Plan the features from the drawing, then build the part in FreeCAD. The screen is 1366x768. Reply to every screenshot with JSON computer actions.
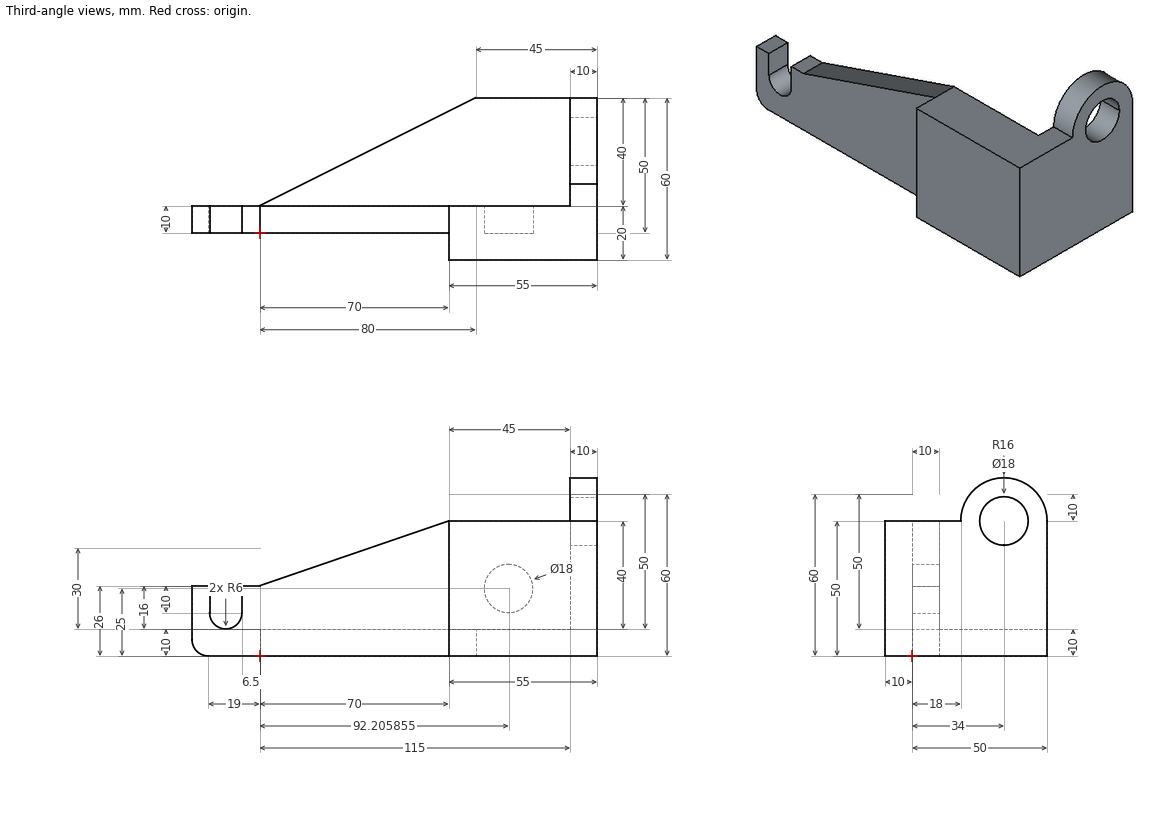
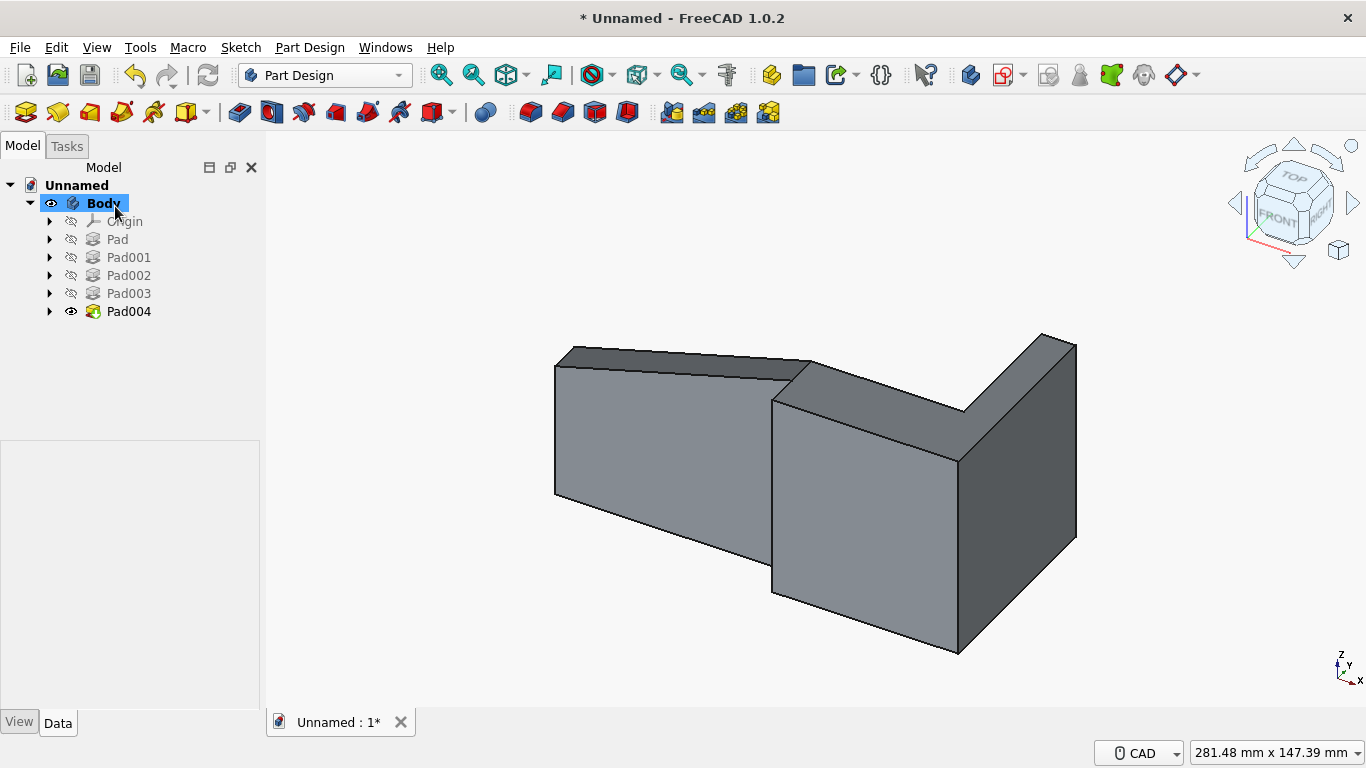
{"action": "left_click", "coordinate": [944, 423]}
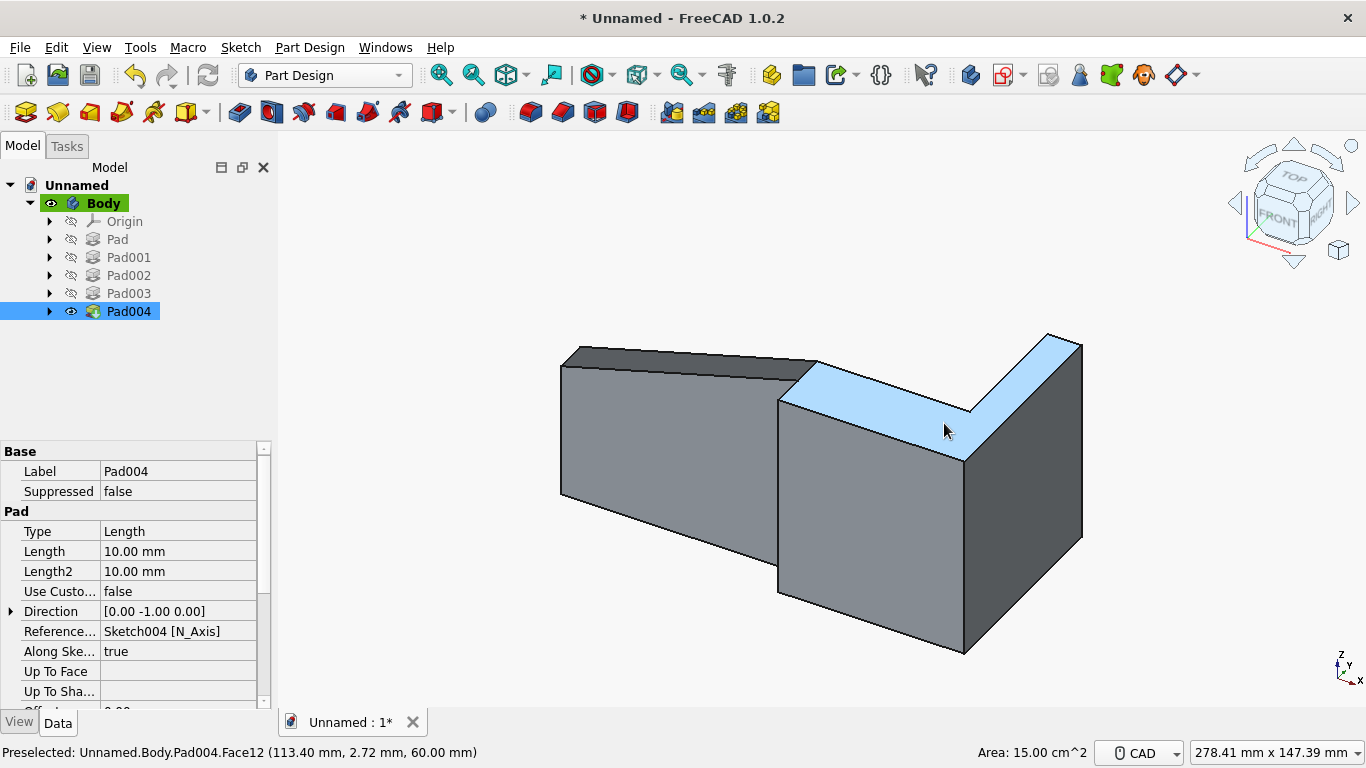
{"action": "left_click", "coordinate": [1004, 76]}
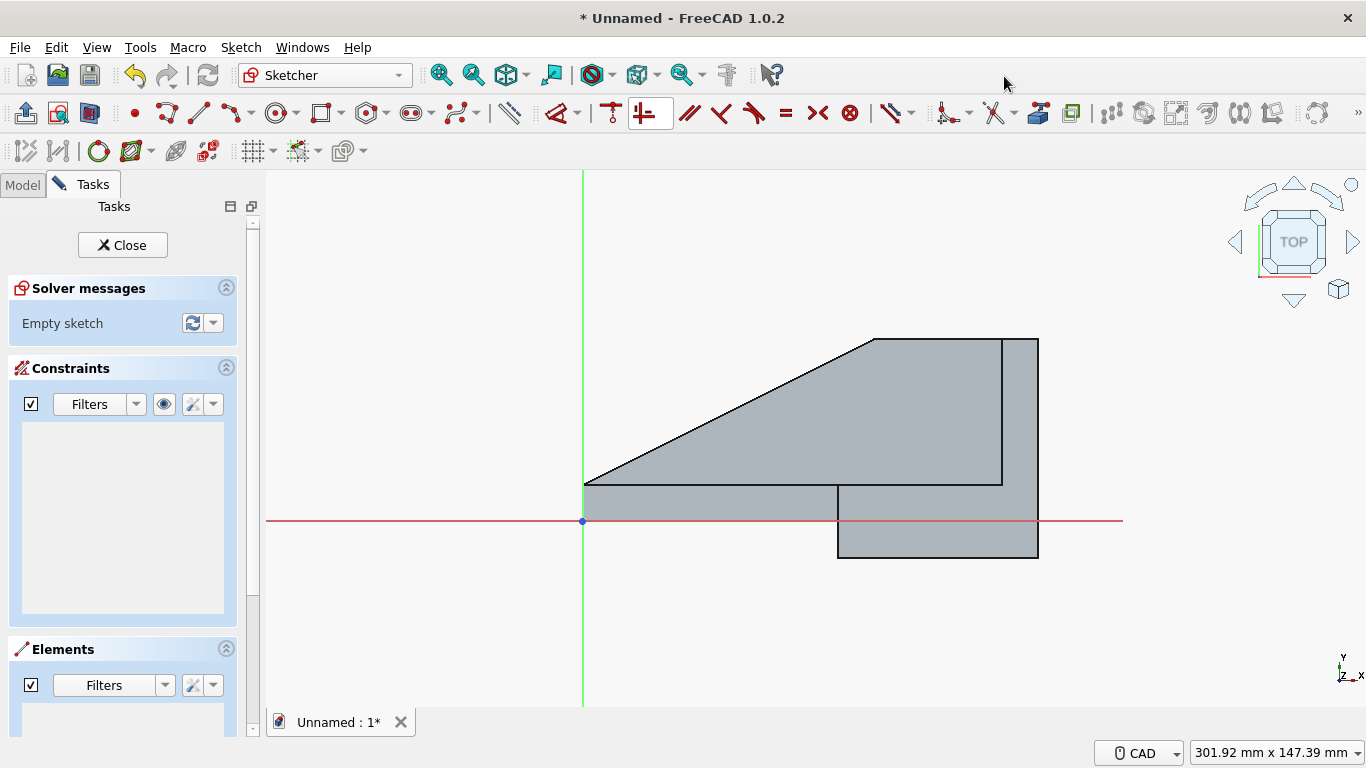
{"action": "scroll", "coordinate": [938, 469], "scroll_direction": "up", "scroll_amount": 2}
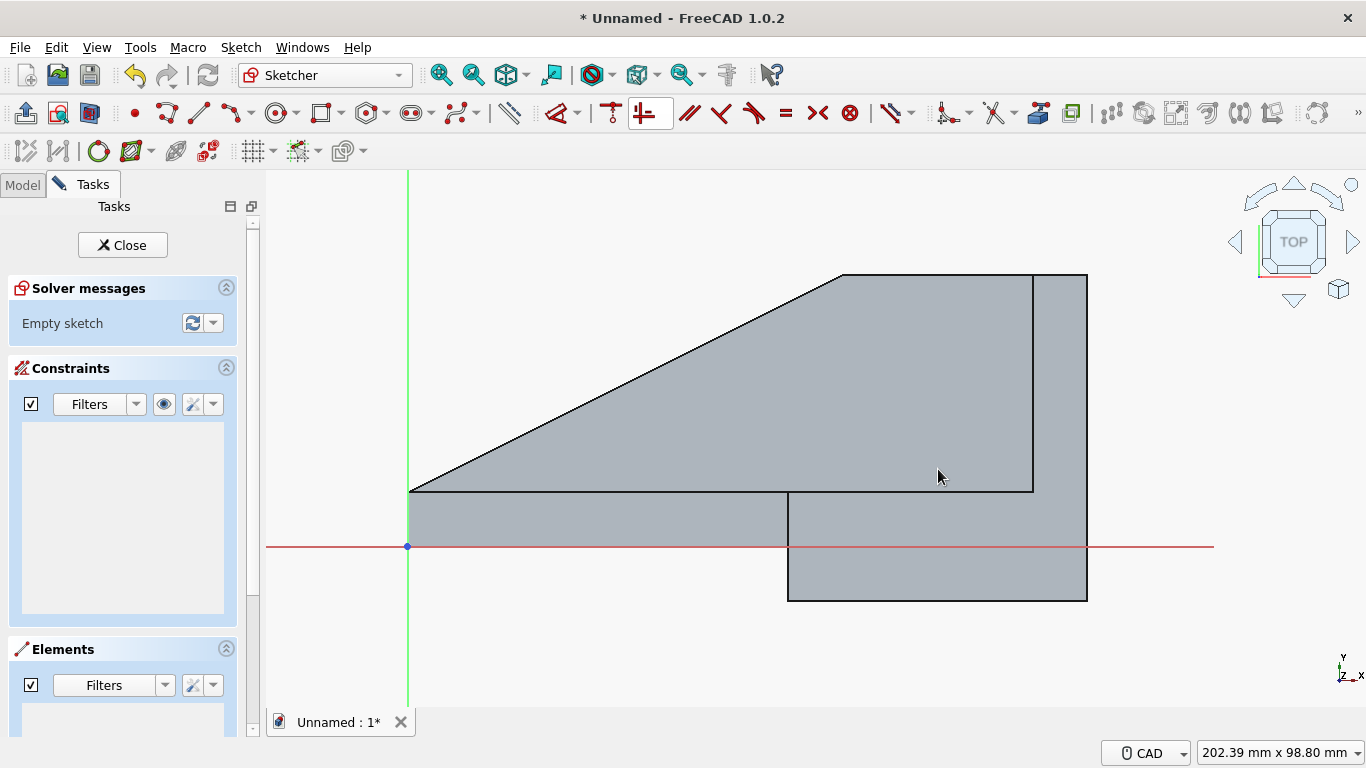
{"action": "left_click", "coordinate": [168, 114]}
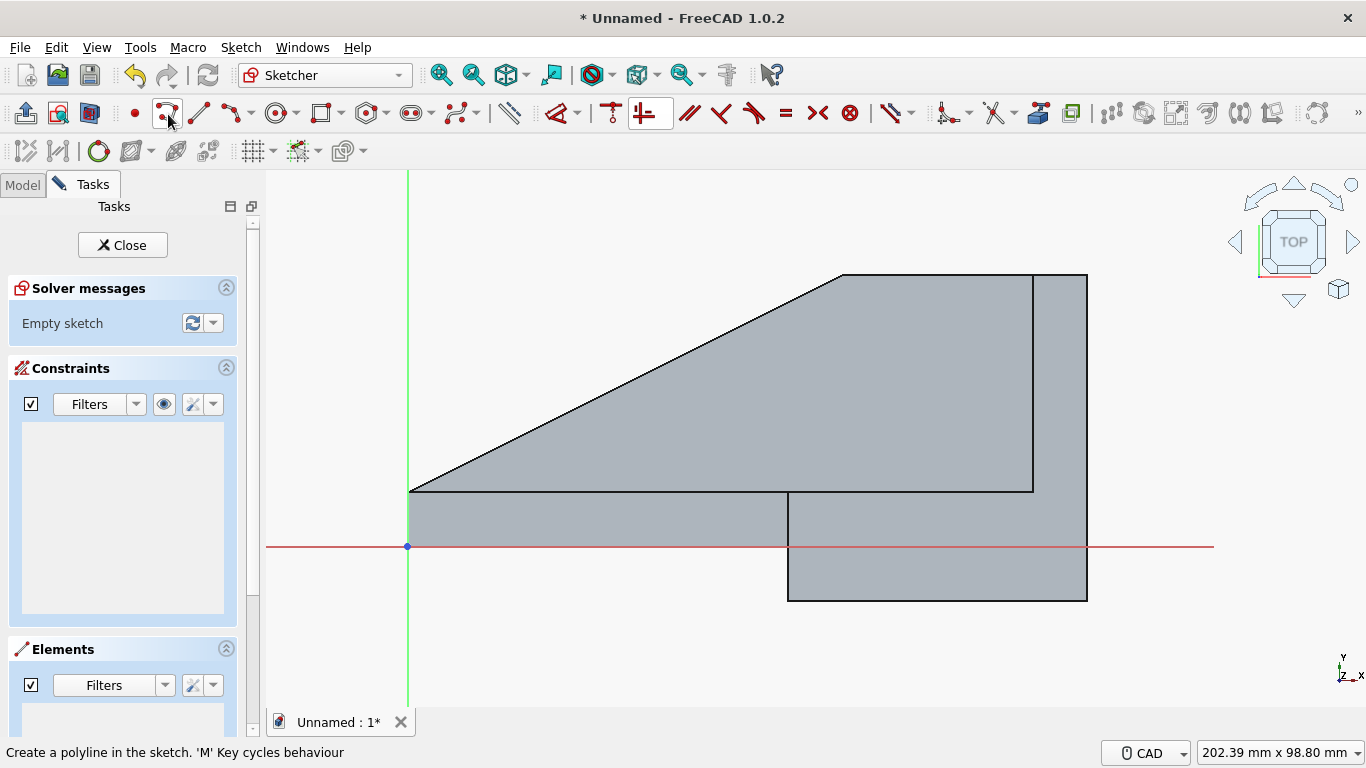
{"action": "left_click", "coordinate": [788, 492]}
{"action": "left_click", "coordinate": [788, 601]}
{"action": "left_click", "coordinate": [1087, 601]}
{"action": "left_click", "coordinate": [1087, 275]}
{"action": "left_click", "coordinate": [1033, 275]}
{"action": "left_click", "coordinate": [1033, 492]}
{"action": "left_click", "coordinate": [788, 493]}
{"action": "key", "text": "Escape"}
{"action": "key", "text": "Escape"}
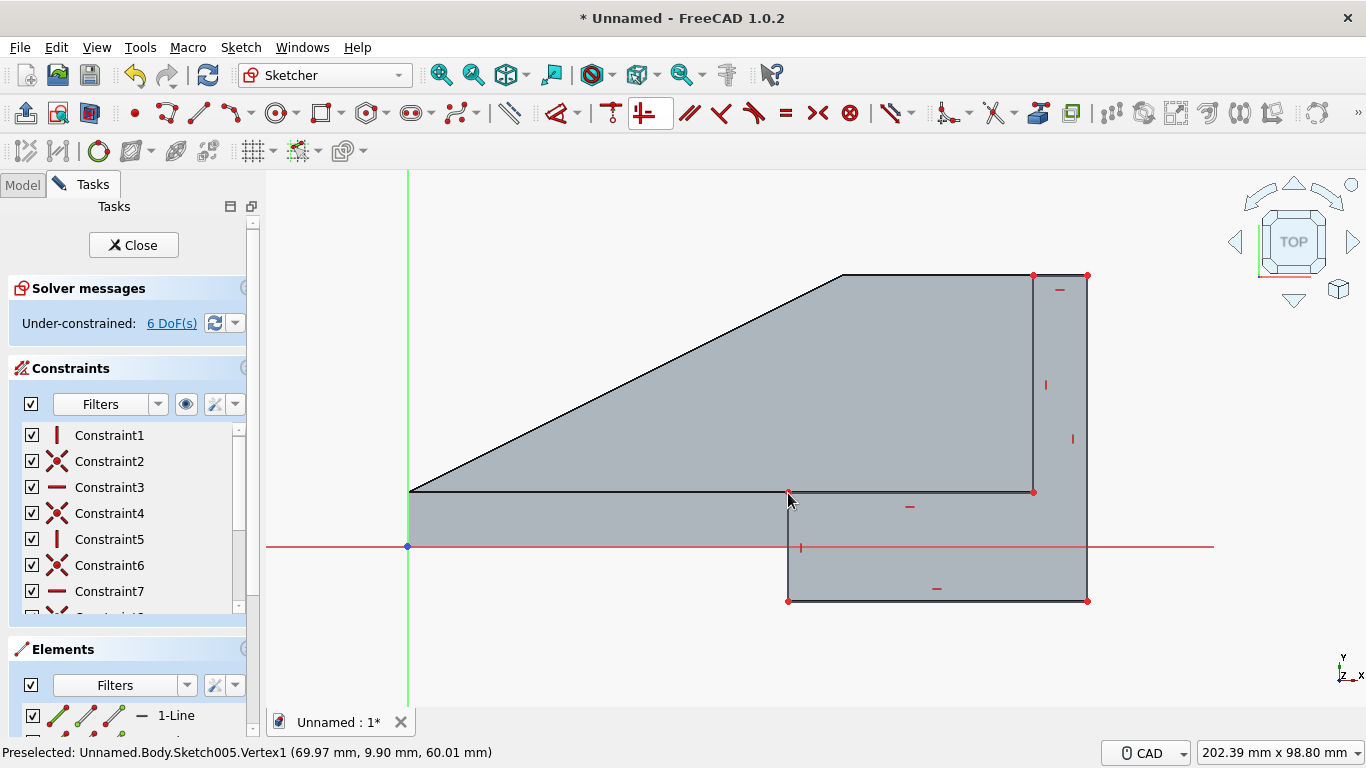
{"action": "left_click", "coordinate": [556, 114]}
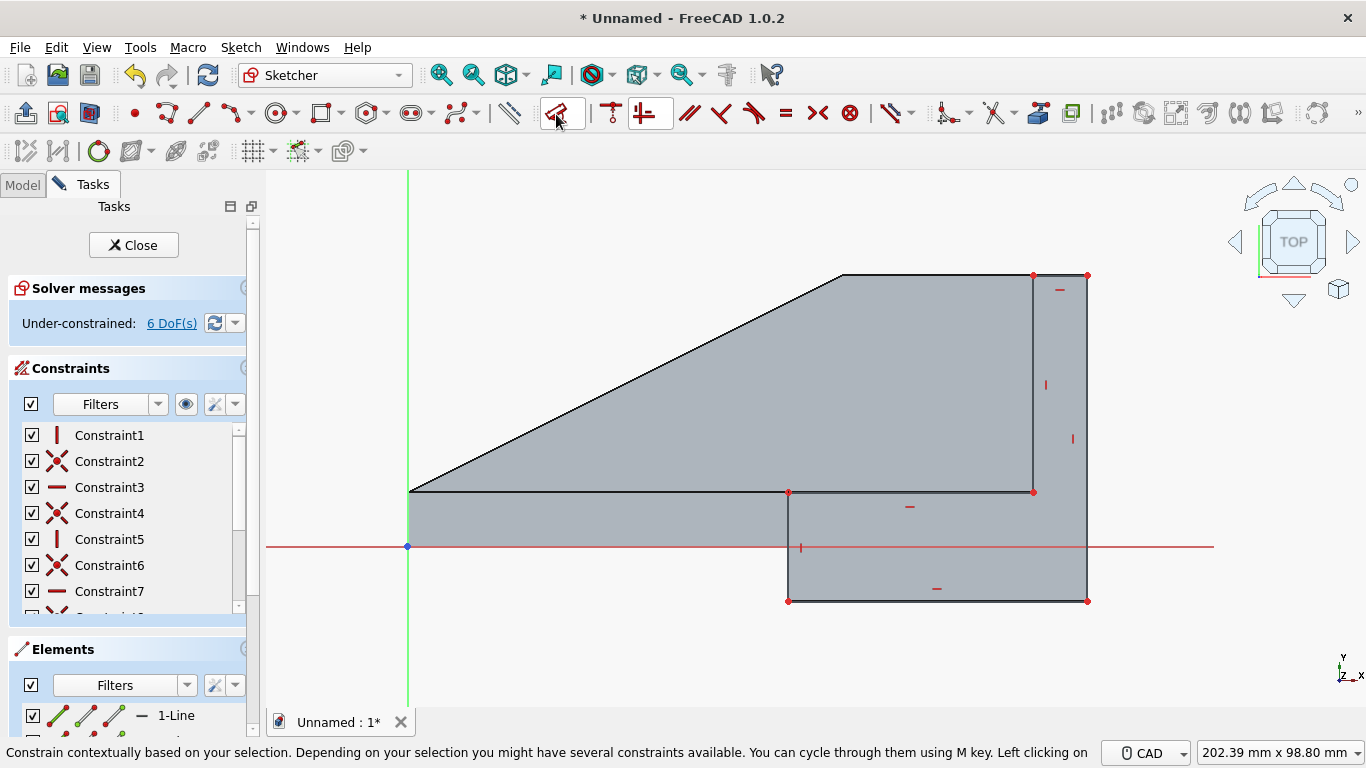
{"action": "left_click", "coordinate": [788, 526]}
{"action": "left_click", "coordinate": [822, 522]}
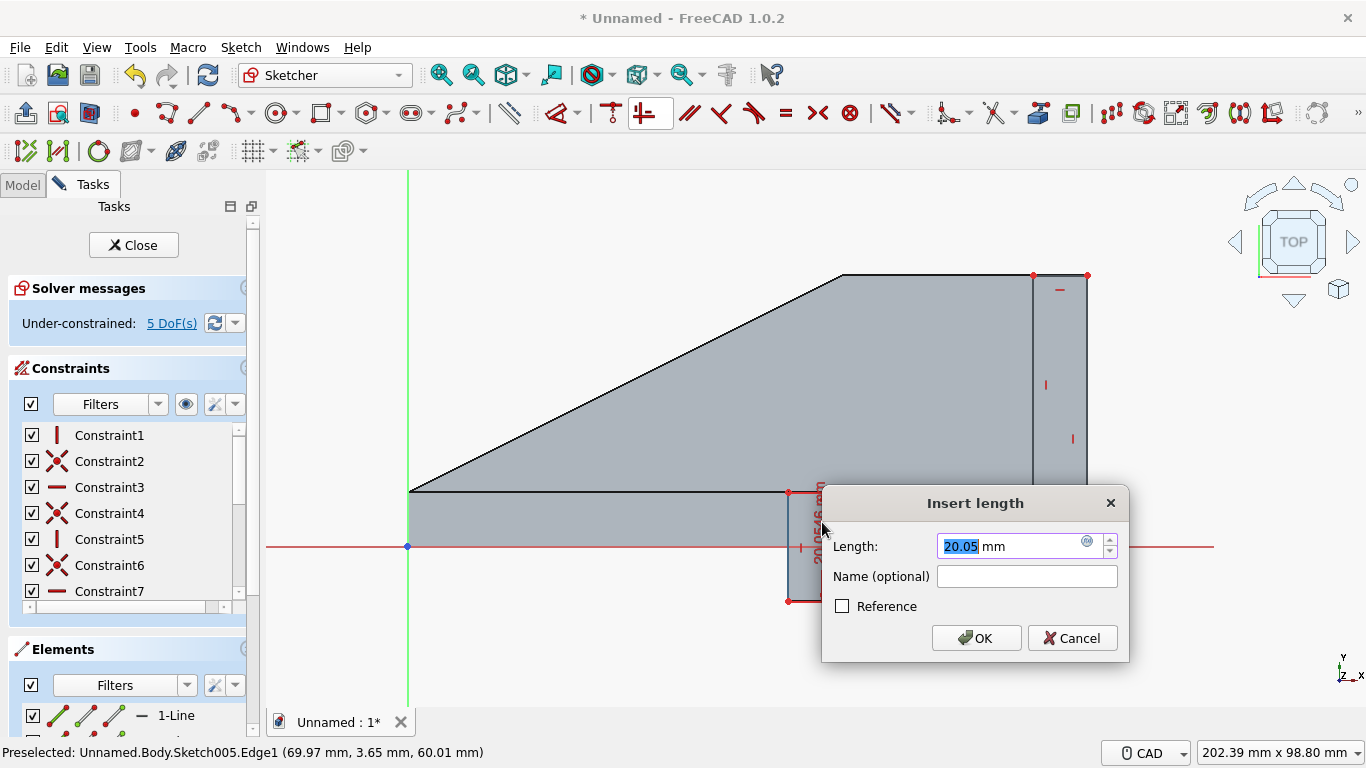
{"action": "type", "text": "20"}
{"action": "key", "text": "Return"}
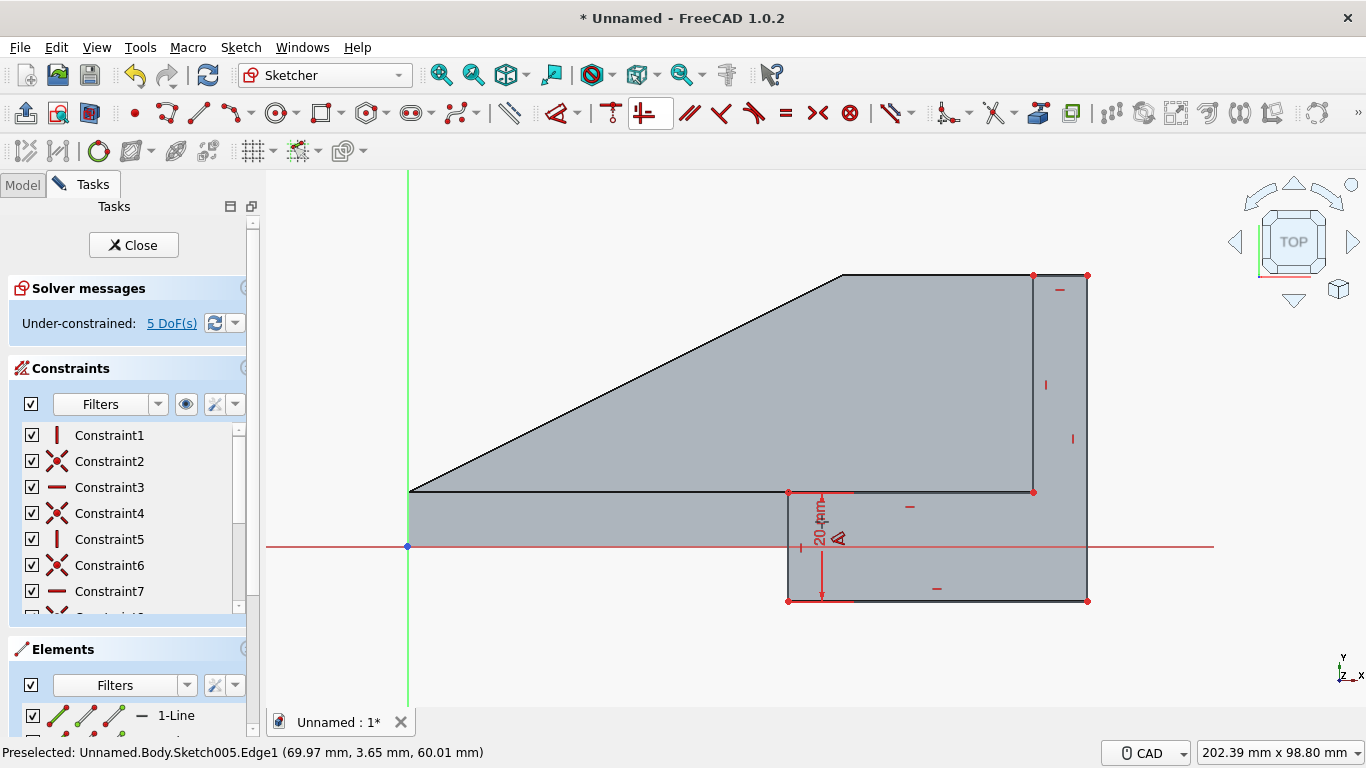
{"action": "left_click", "coordinate": [878, 602]}
{"action": "left_click", "coordinate": [937, 636]}